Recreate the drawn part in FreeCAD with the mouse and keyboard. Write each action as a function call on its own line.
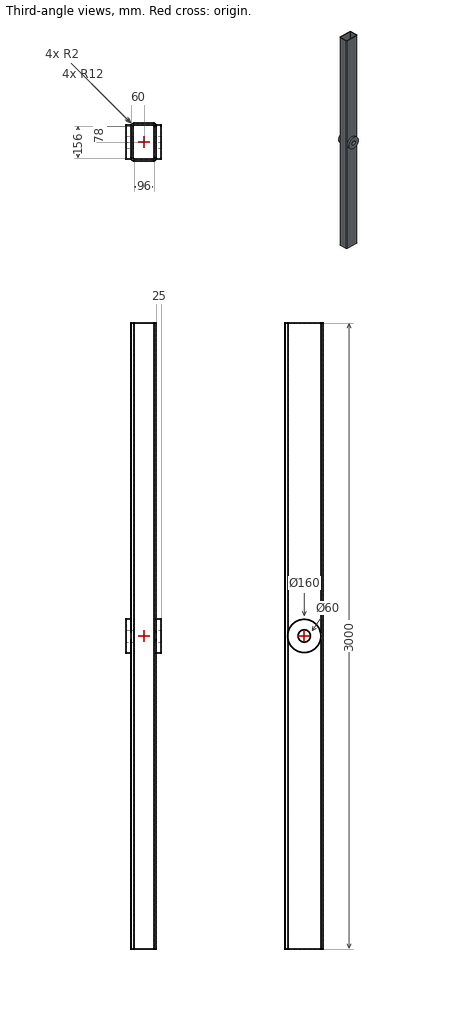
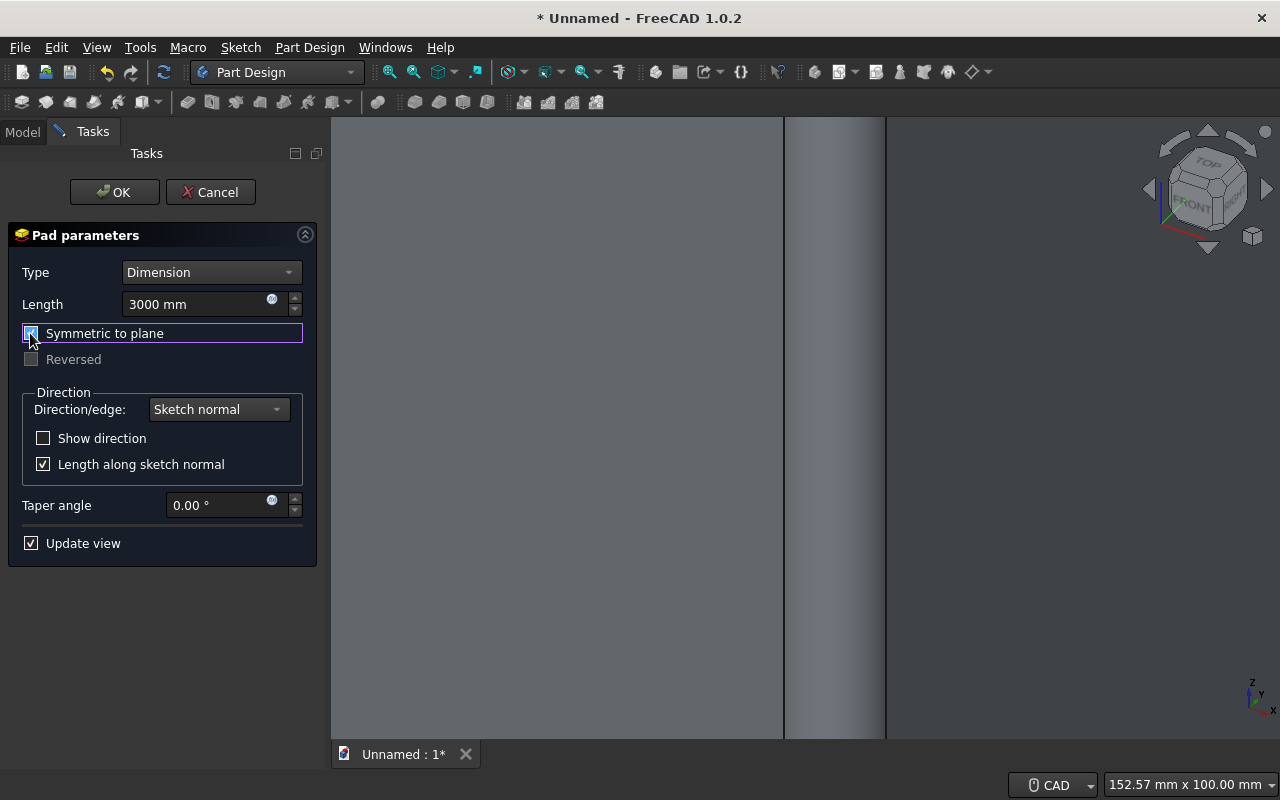
click(115, 192)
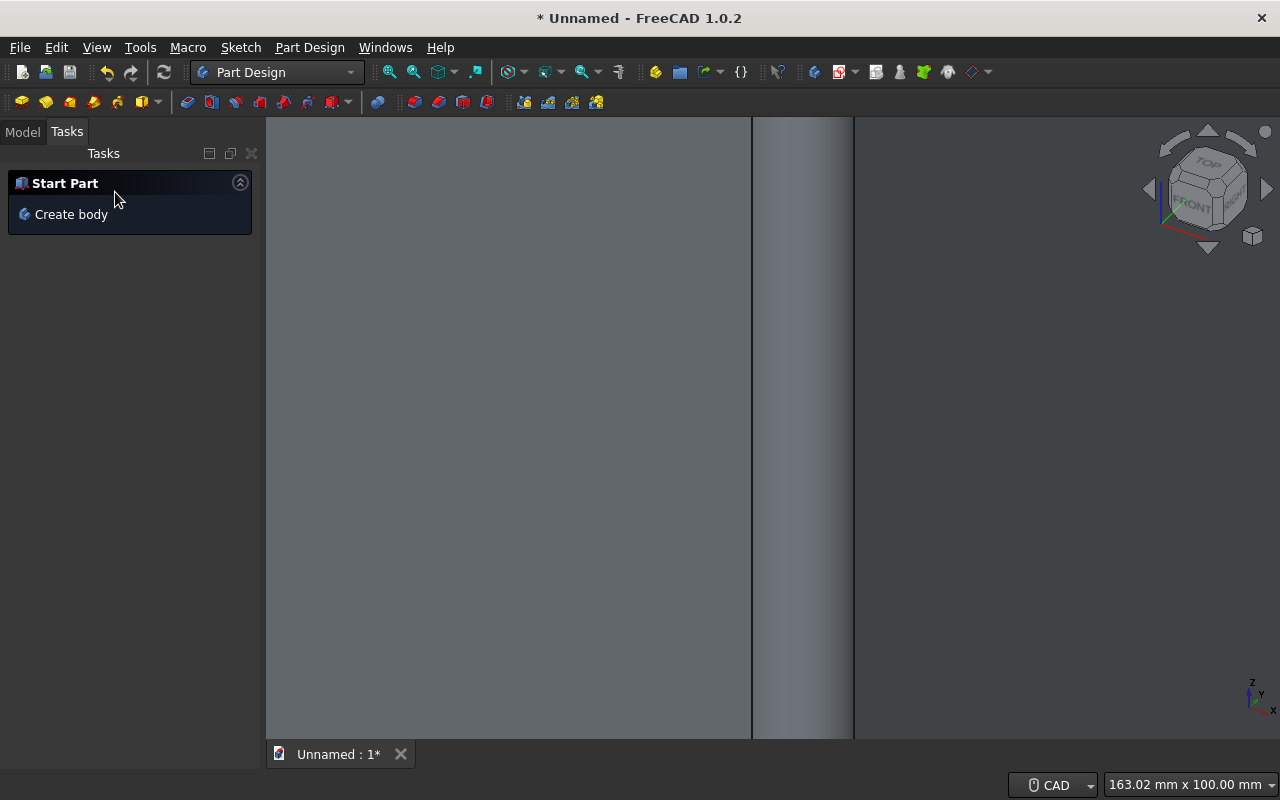
click(390, 72)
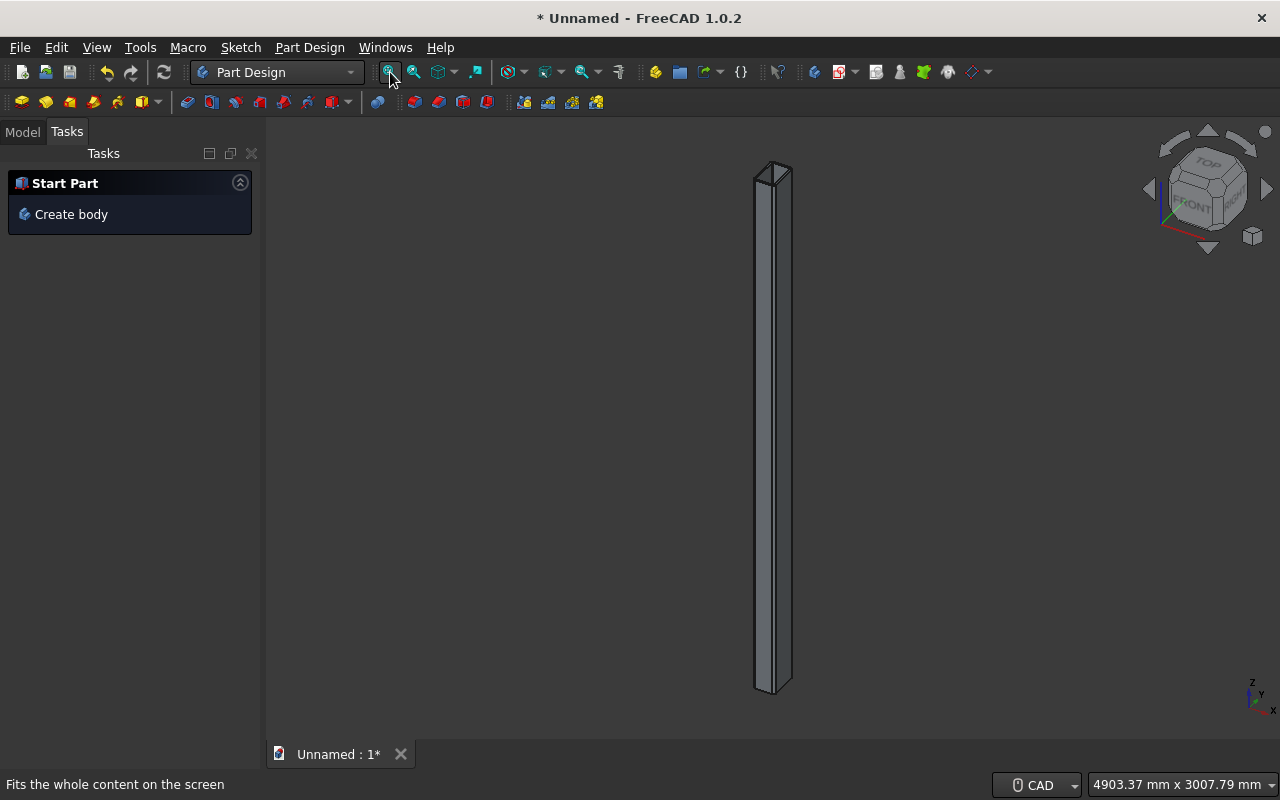
click(840, 72)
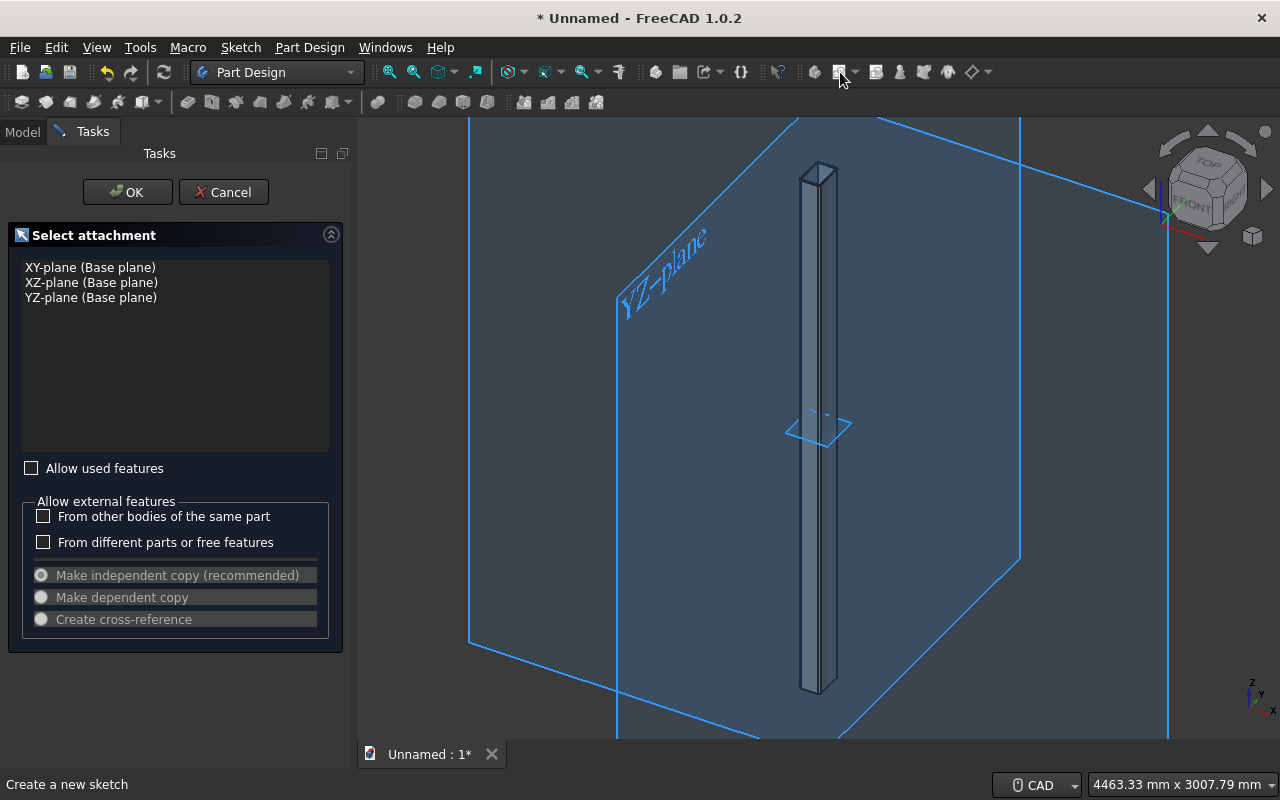
click(82, 298)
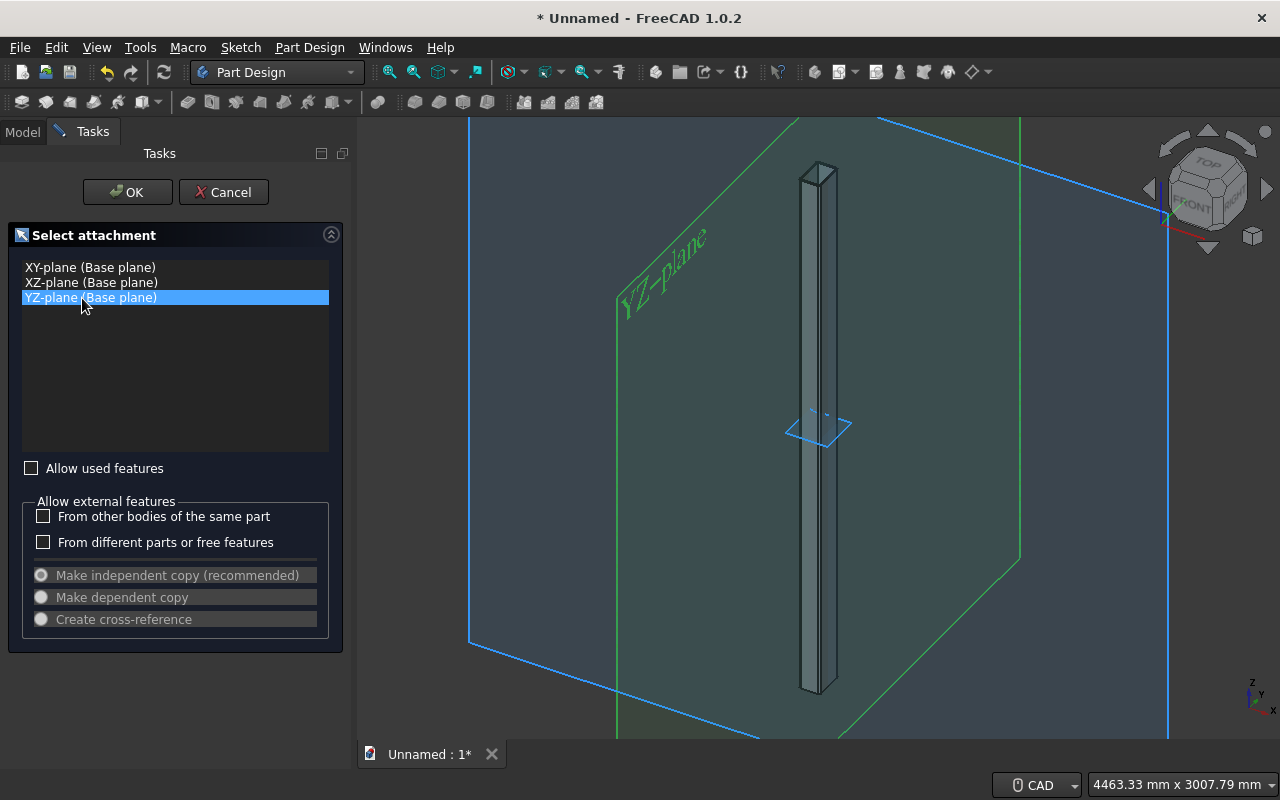
click(128, 192)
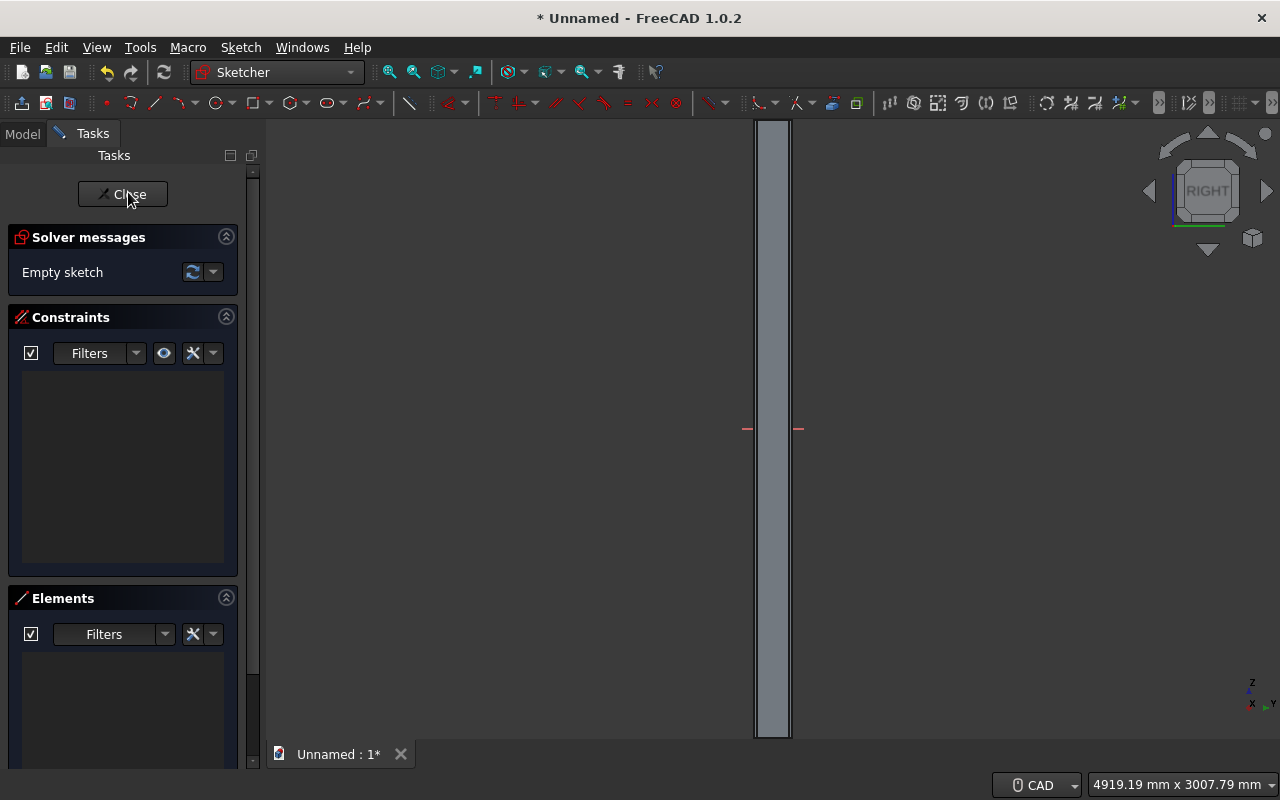
click(70, 104)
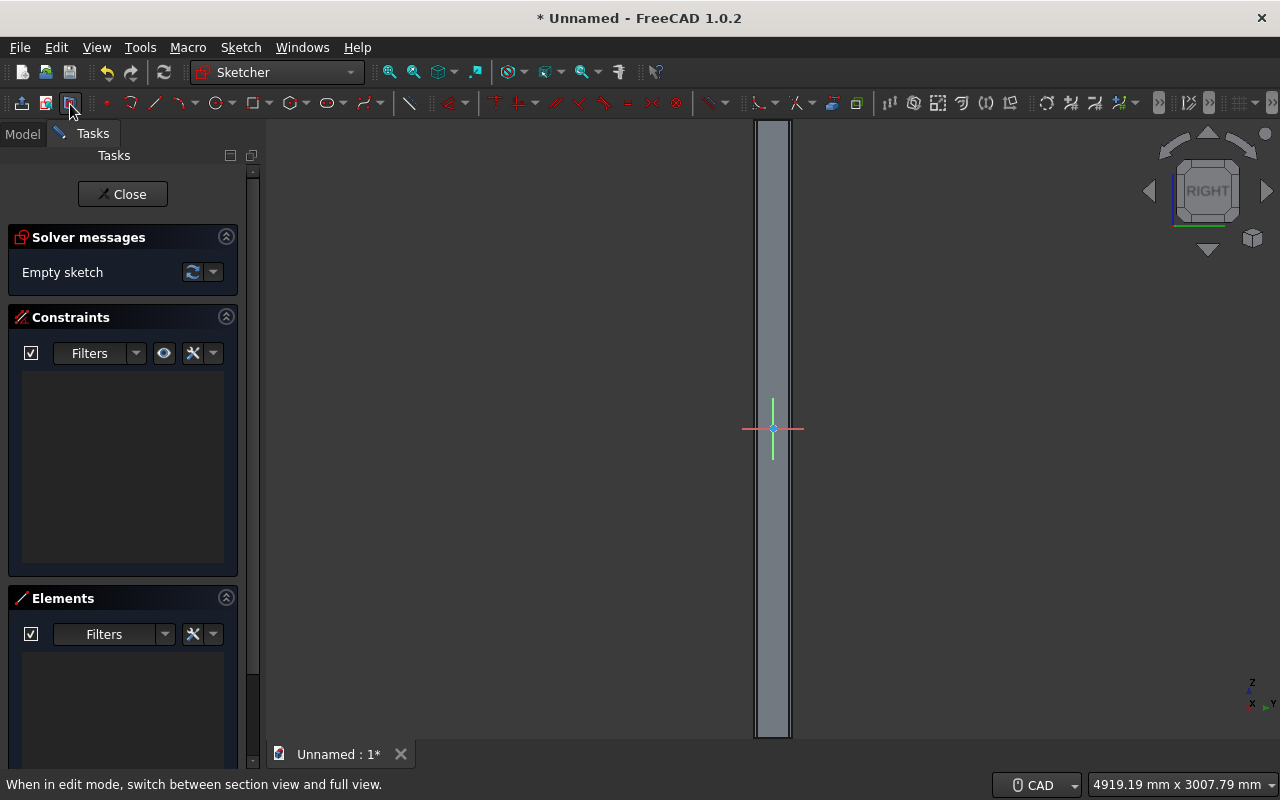
scroll(777, 429, up, 15)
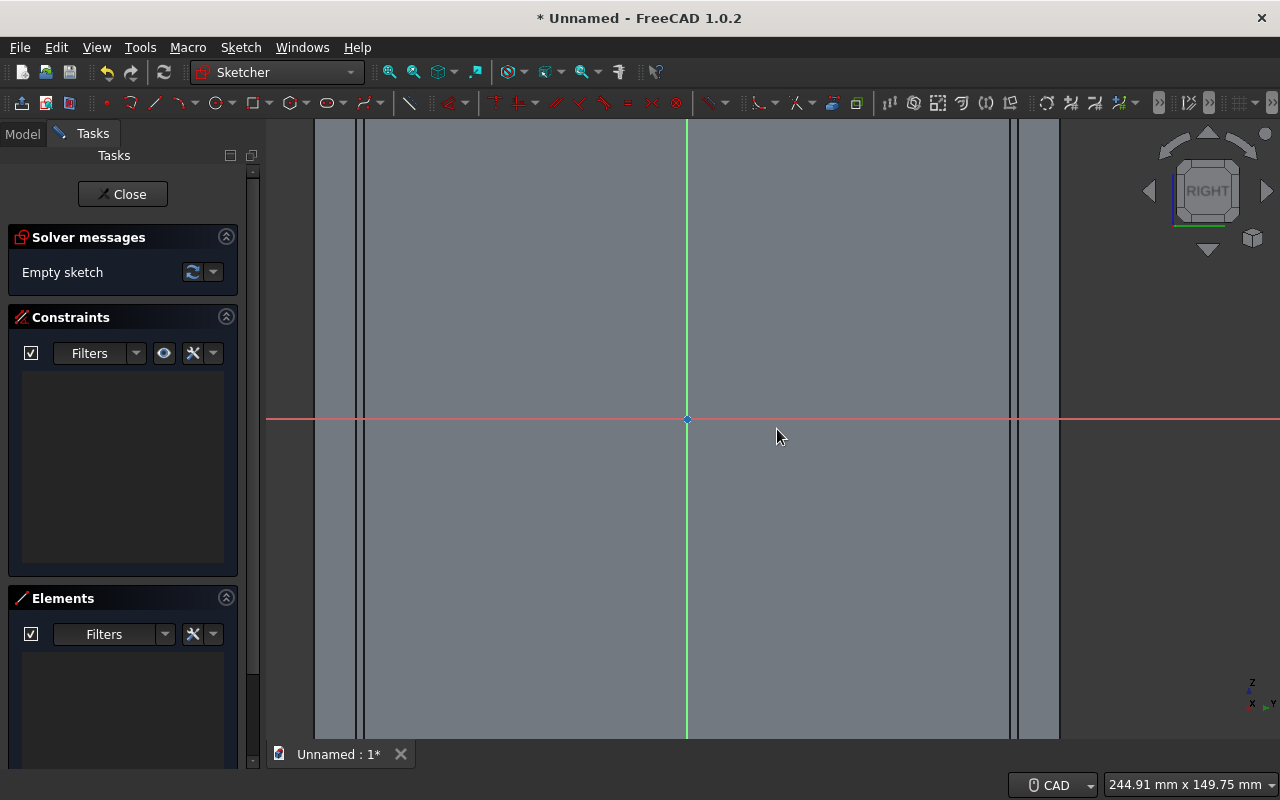
scroll(652, 400, up, 2)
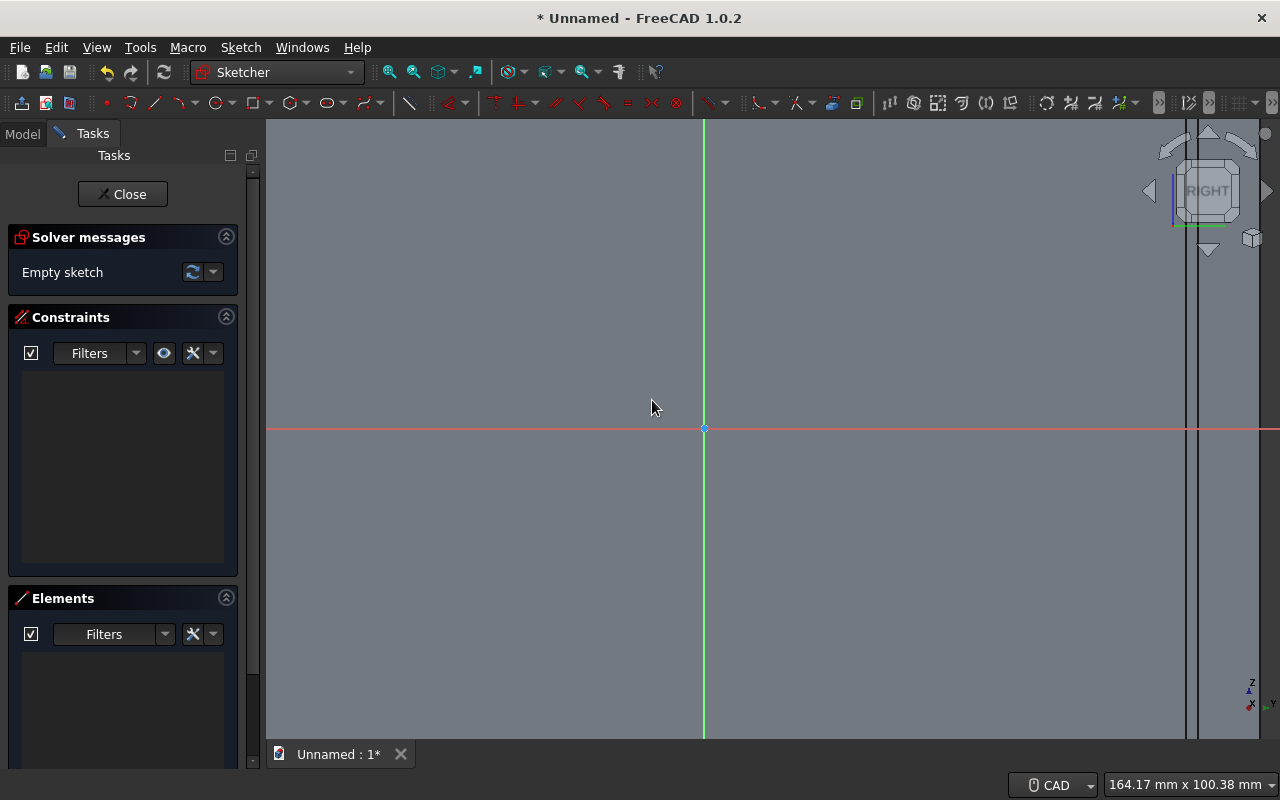
click(216, 104)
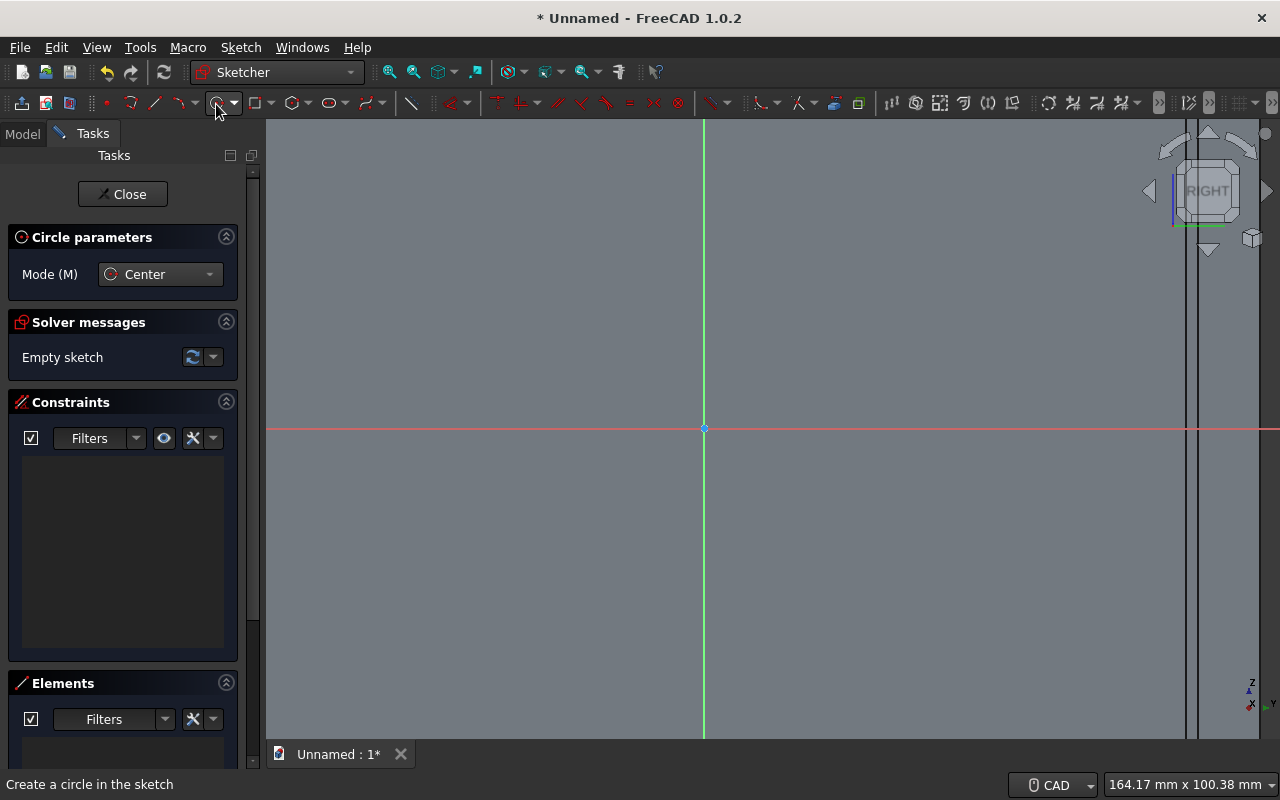
click(704, 429)
click(835, 298)
key(Escape)